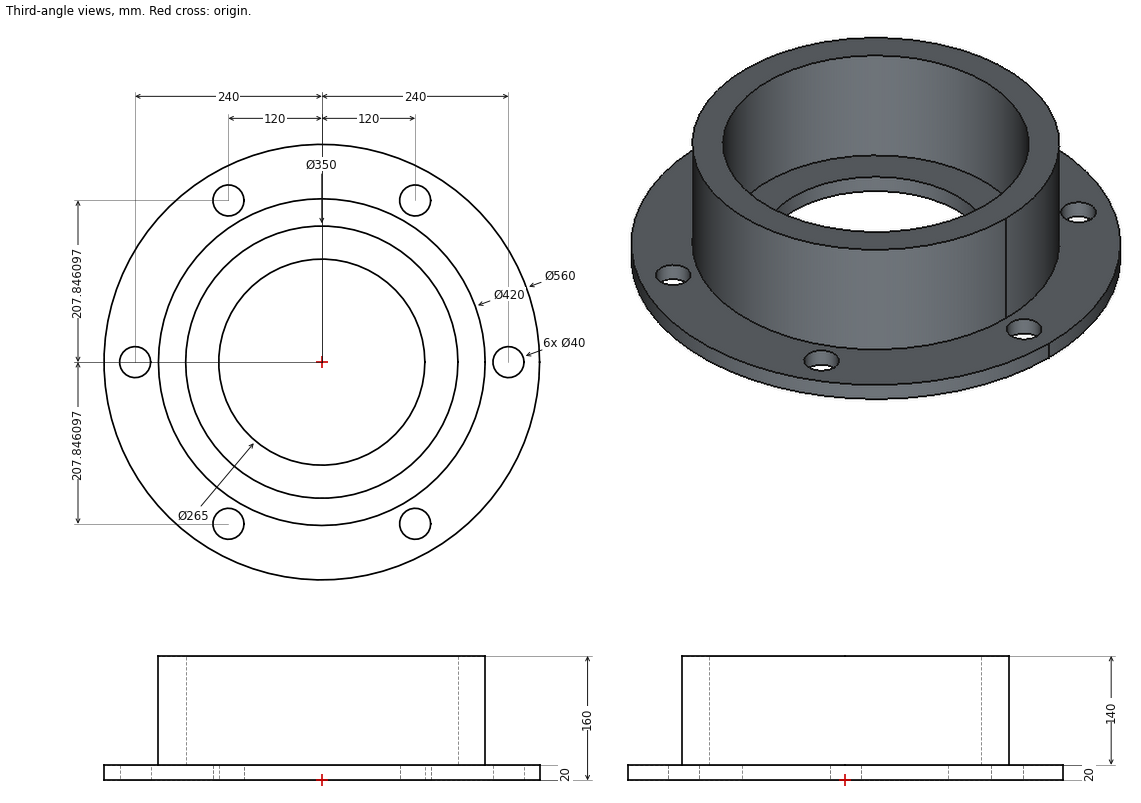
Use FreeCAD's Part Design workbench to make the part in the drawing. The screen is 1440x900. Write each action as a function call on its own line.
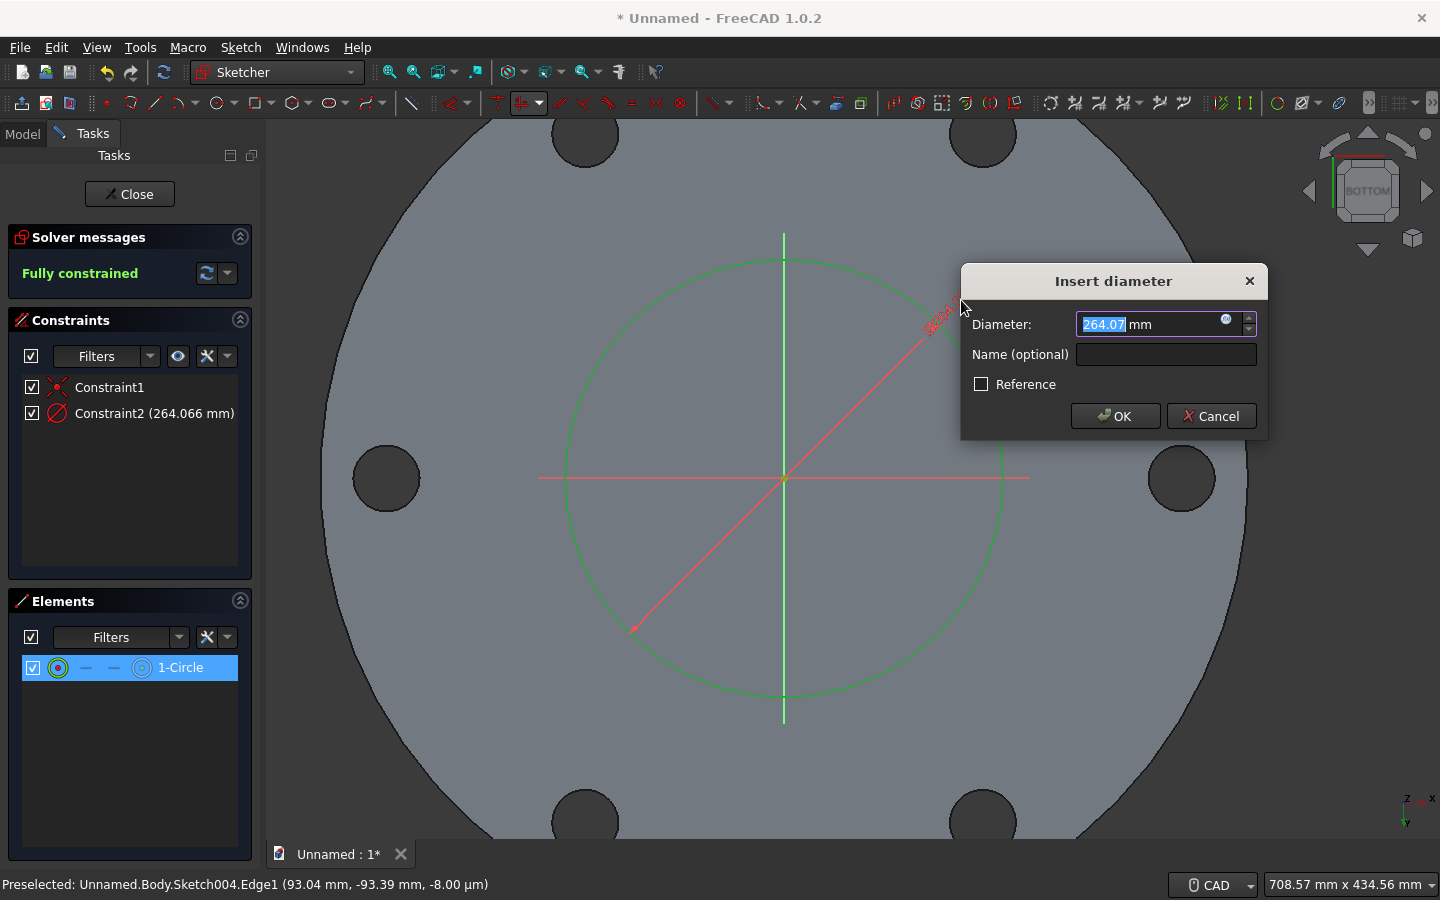
text(265)
key(Return)
key(Escape)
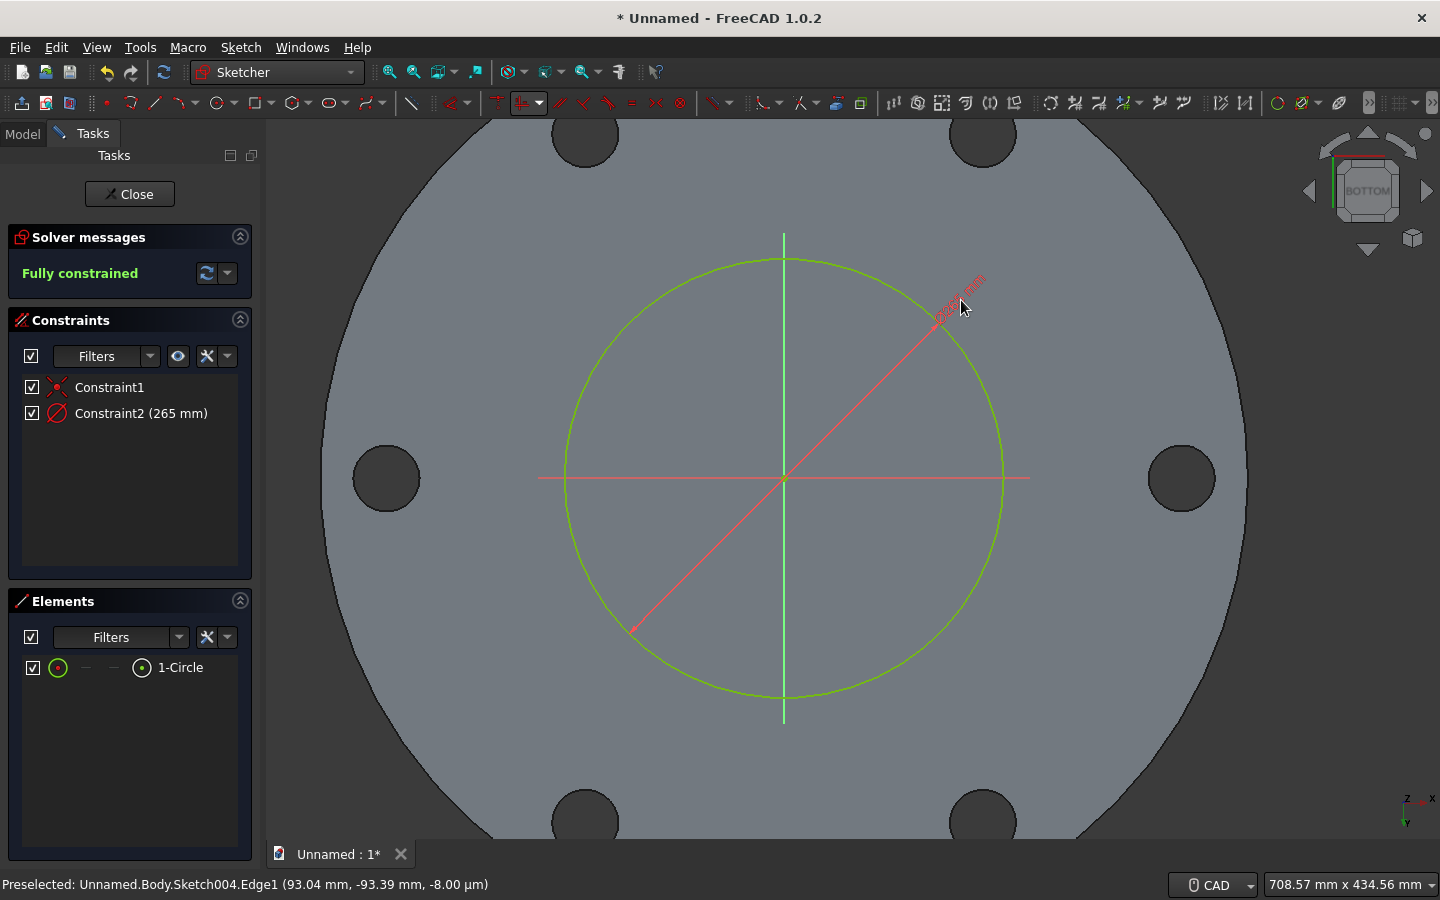
click(130, 194)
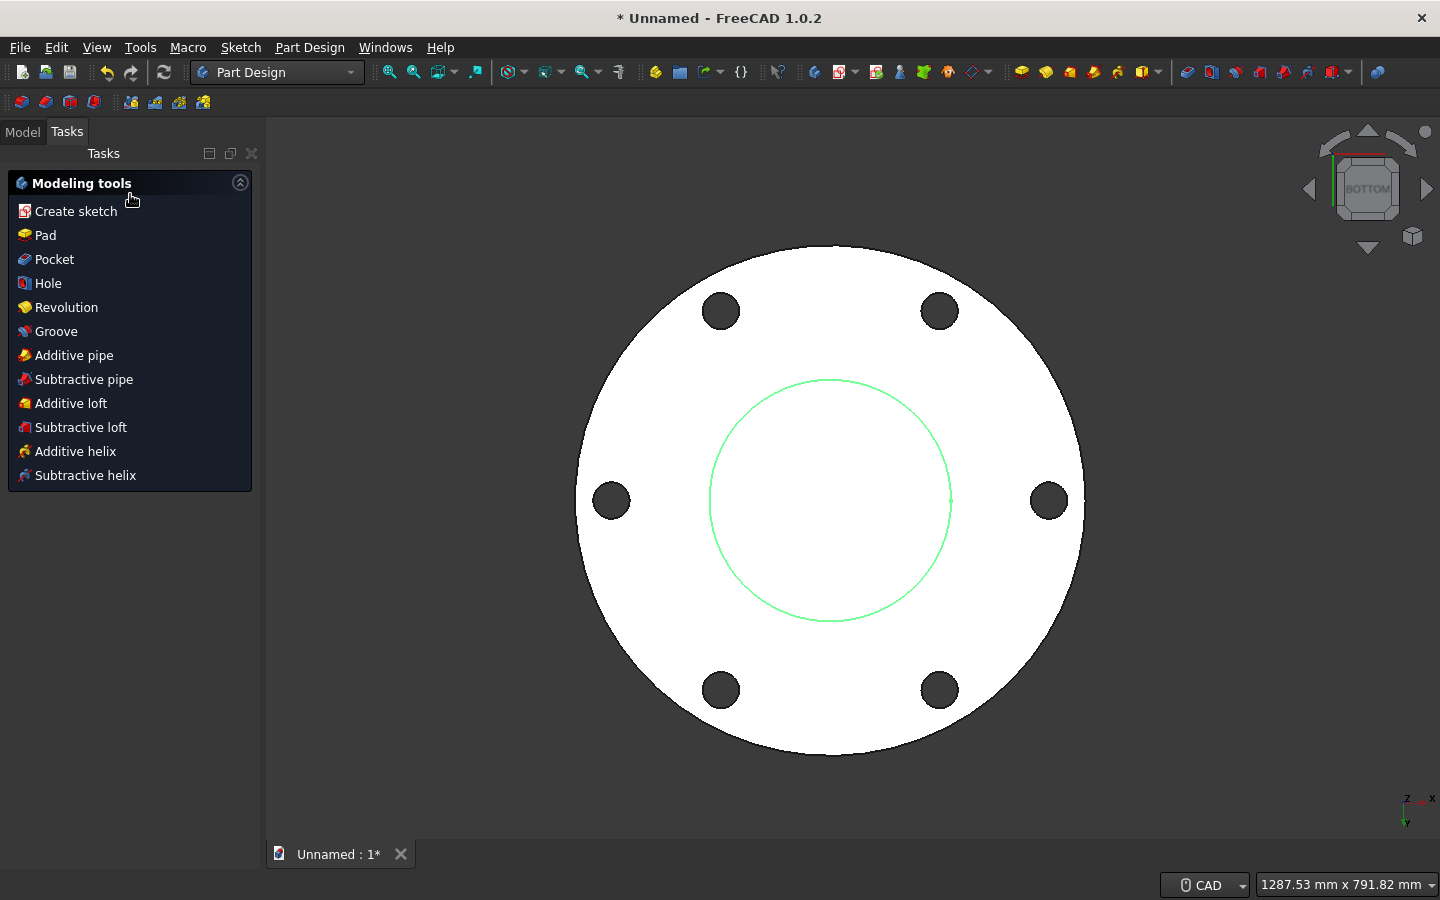
click(1188, 72)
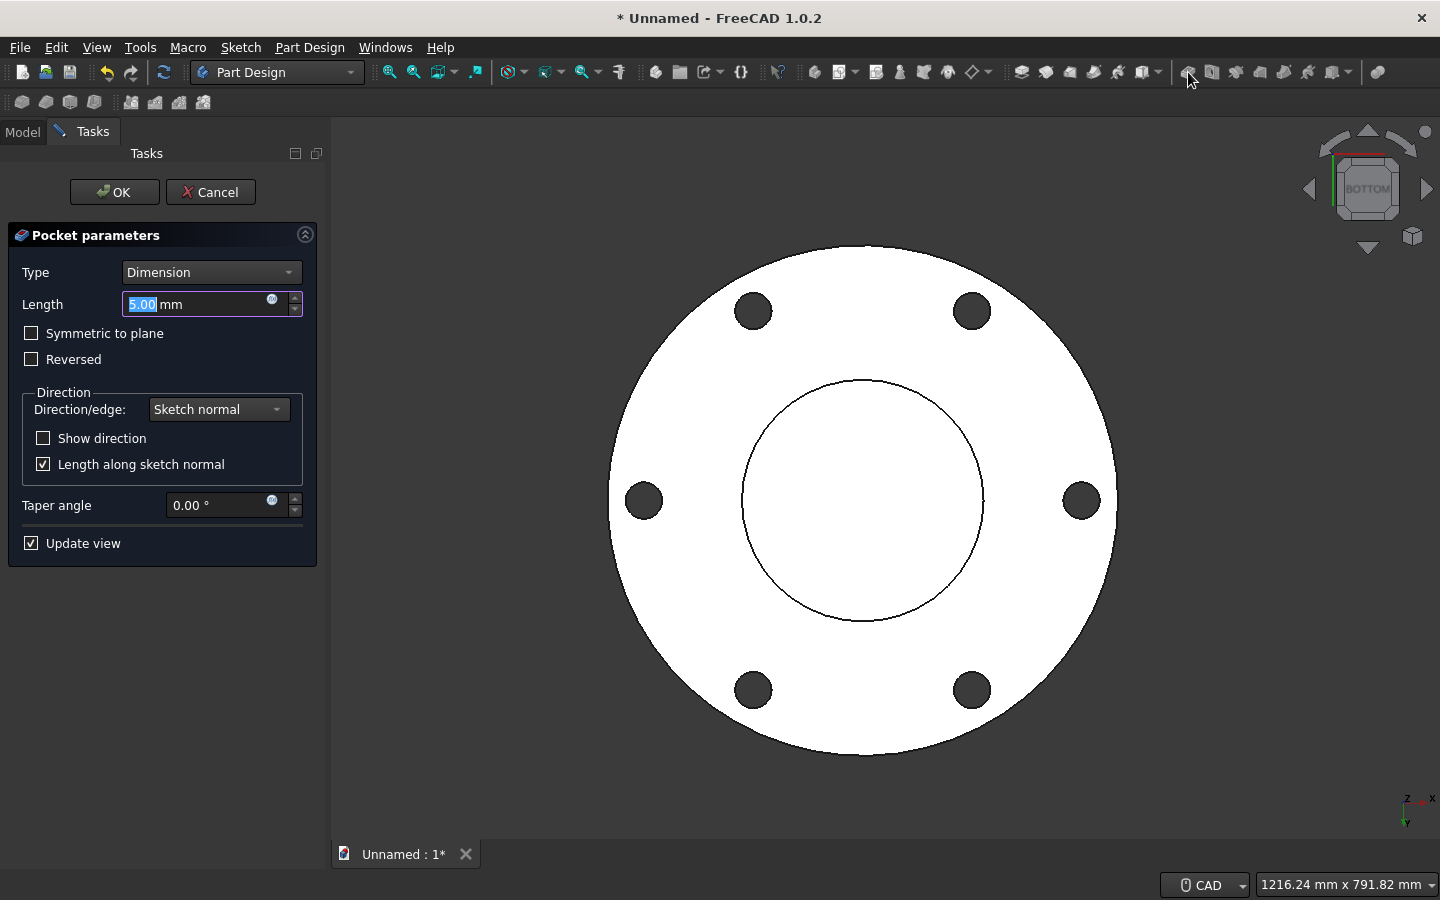
text(20)
key(Tab)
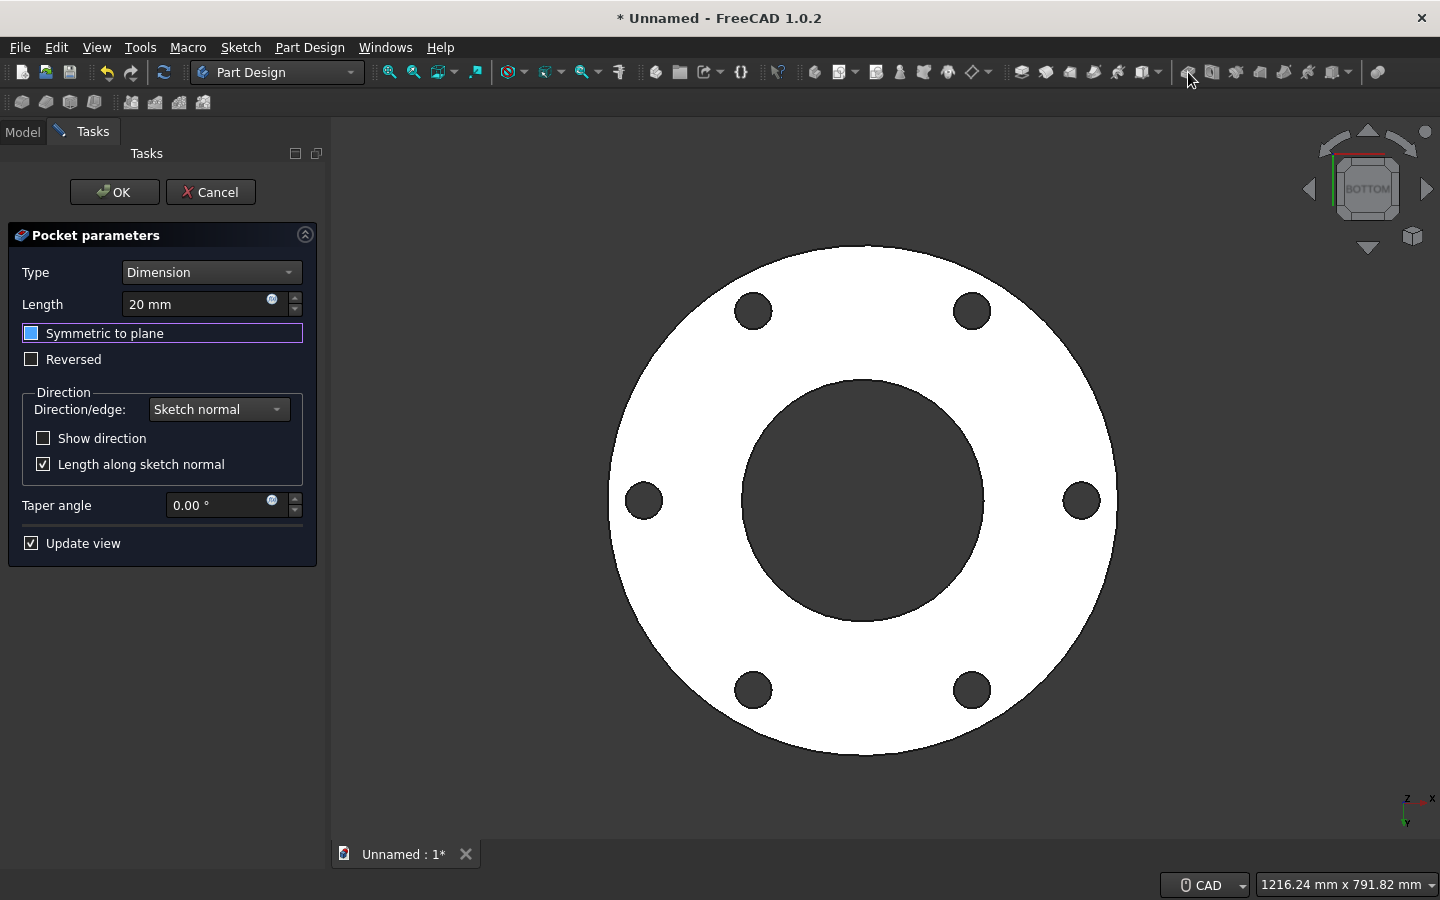
click(115, 192)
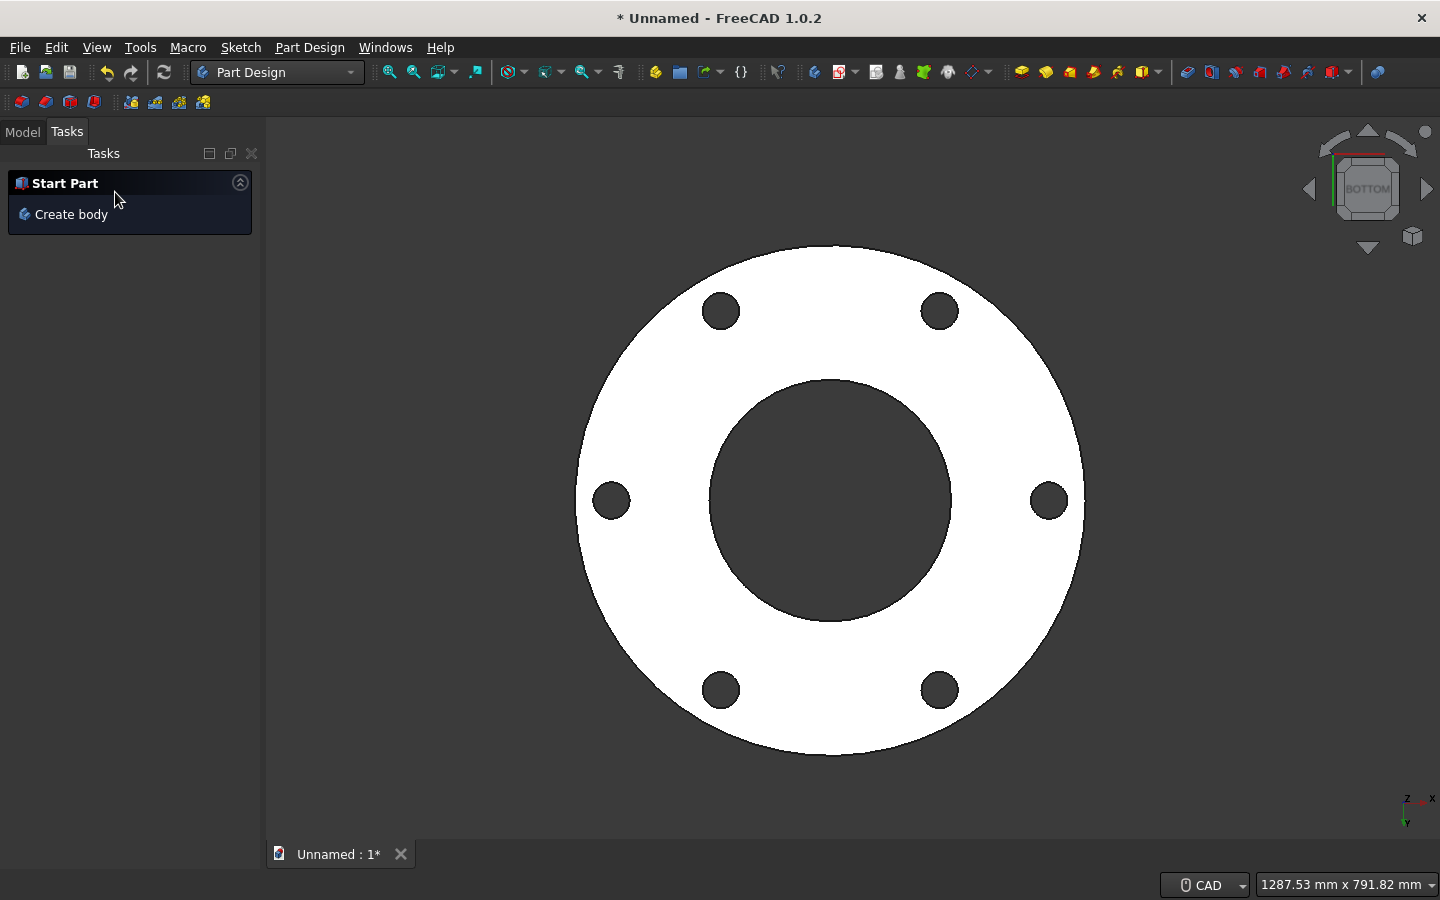
key(0)